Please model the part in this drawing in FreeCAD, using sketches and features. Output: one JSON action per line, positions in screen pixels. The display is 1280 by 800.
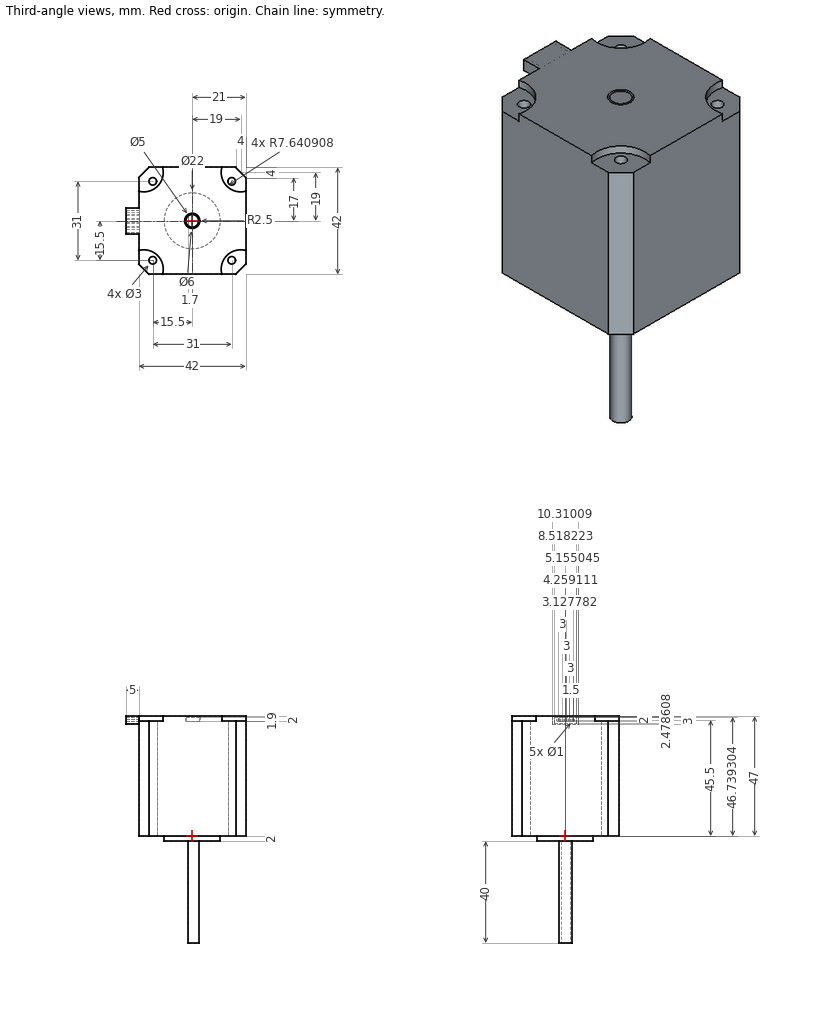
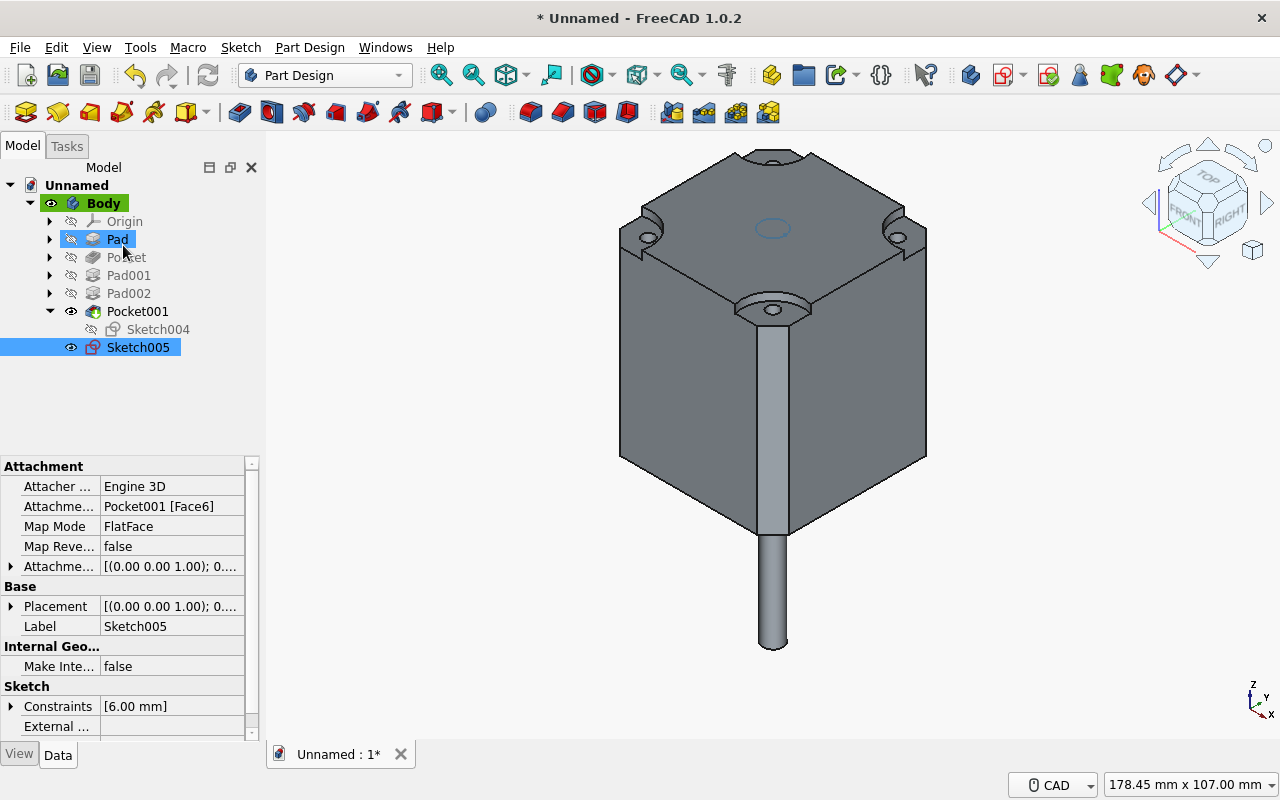
{"action": "left_click", "coordinate": [240, 112]}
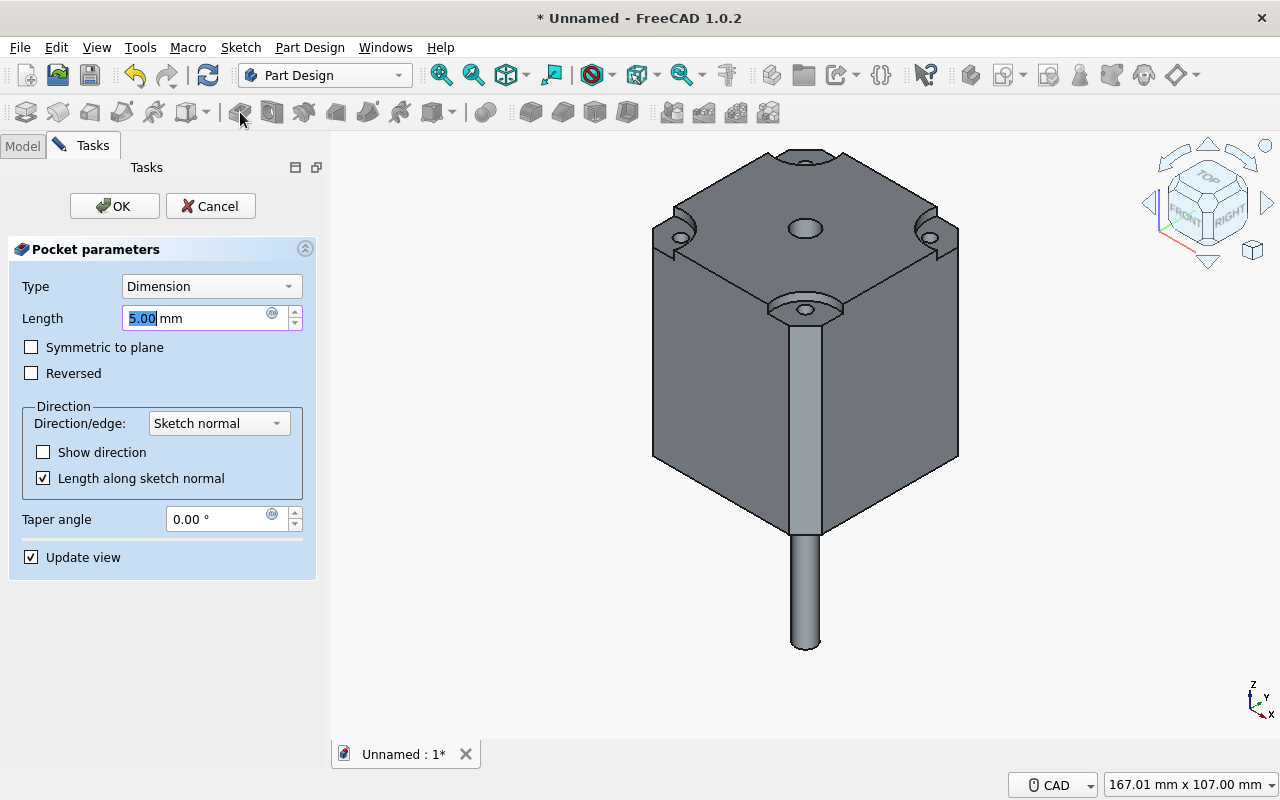
{"action": "type", "text": "2"}
{"action": "key", "text": "Tab"}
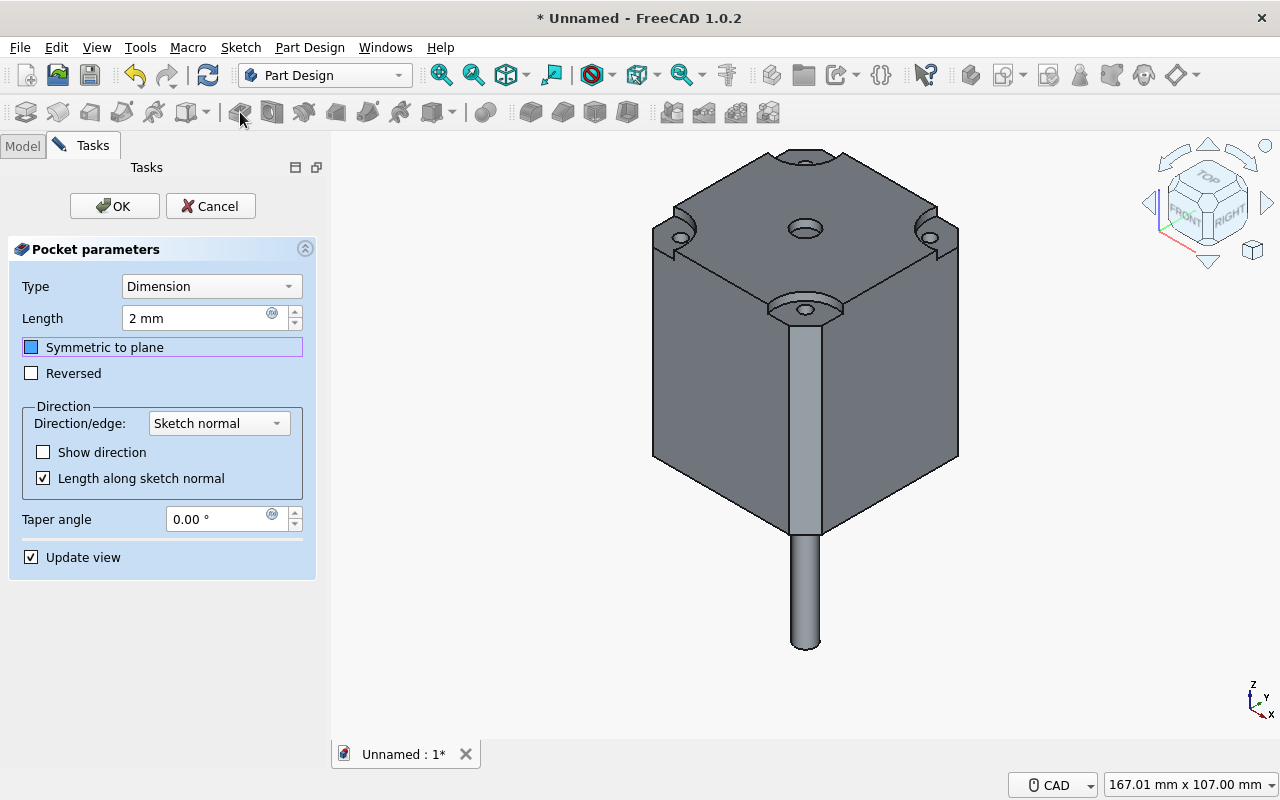
{"action": "left_click", "coordinate": [115, 206]}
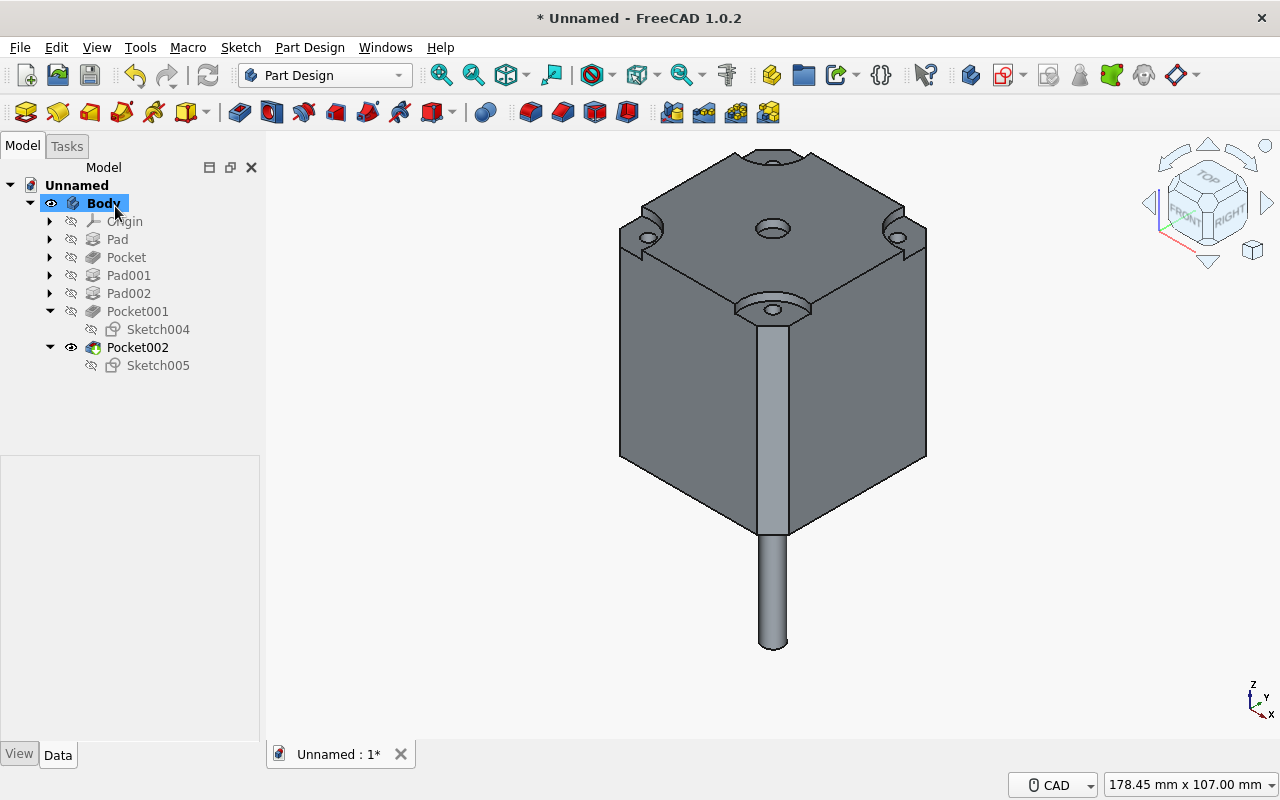
{"action": "left_click", "coordinate": [442, 76]}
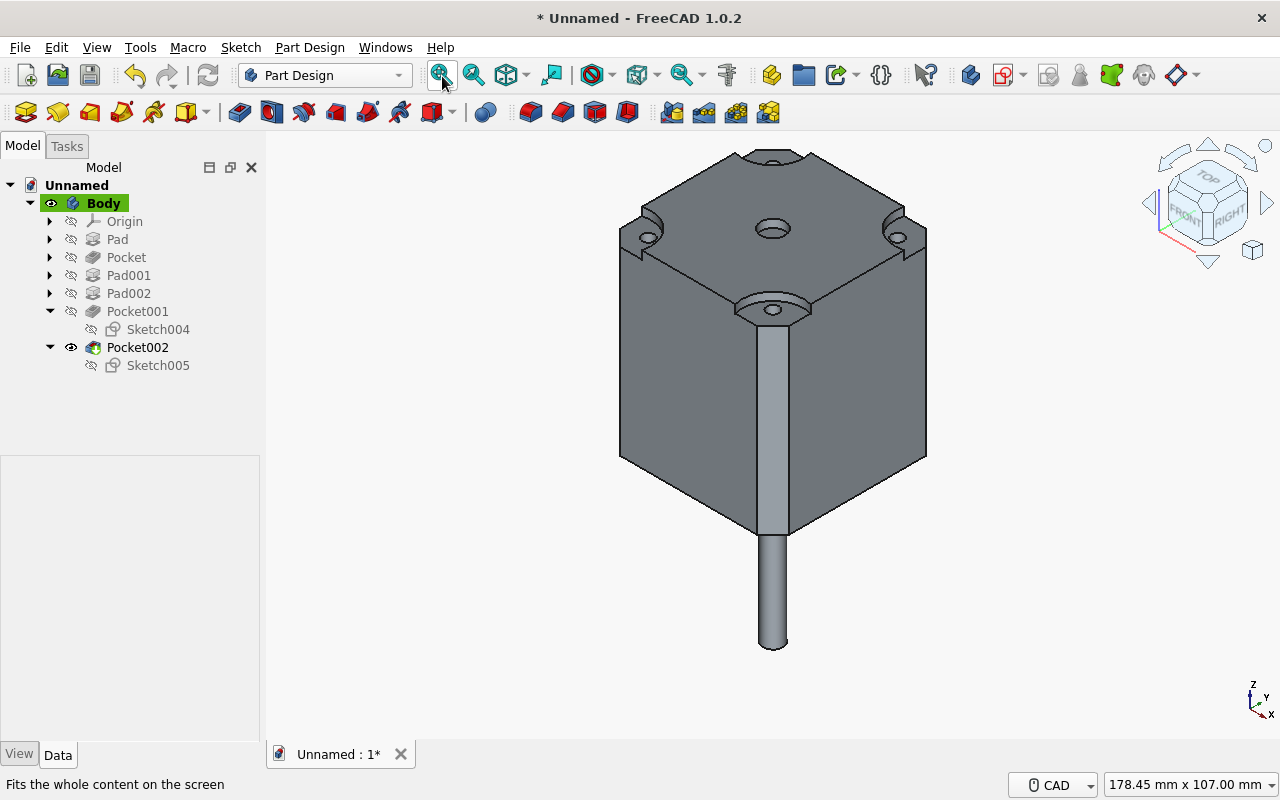
{"action": "left_click", "coordinate": [50, 221]}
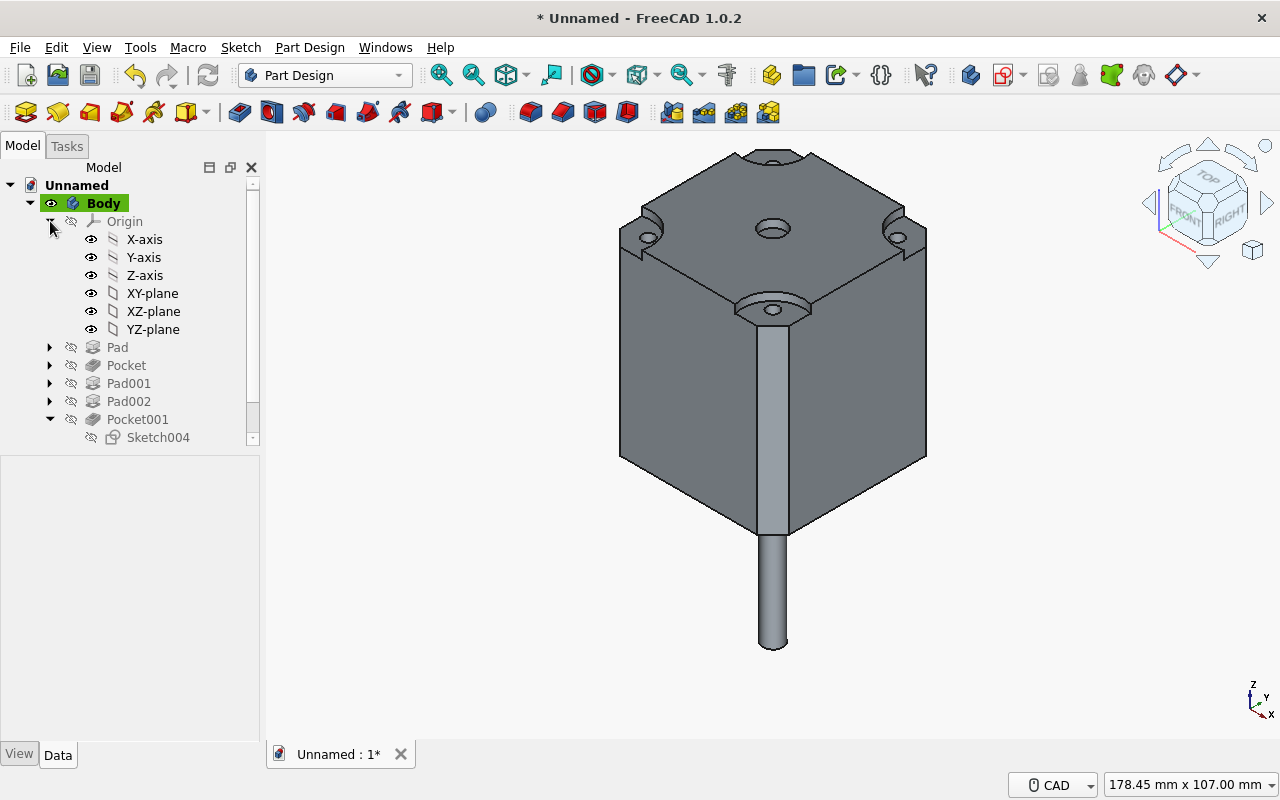
{"action": "left_click", "coordinate": [136, 293]}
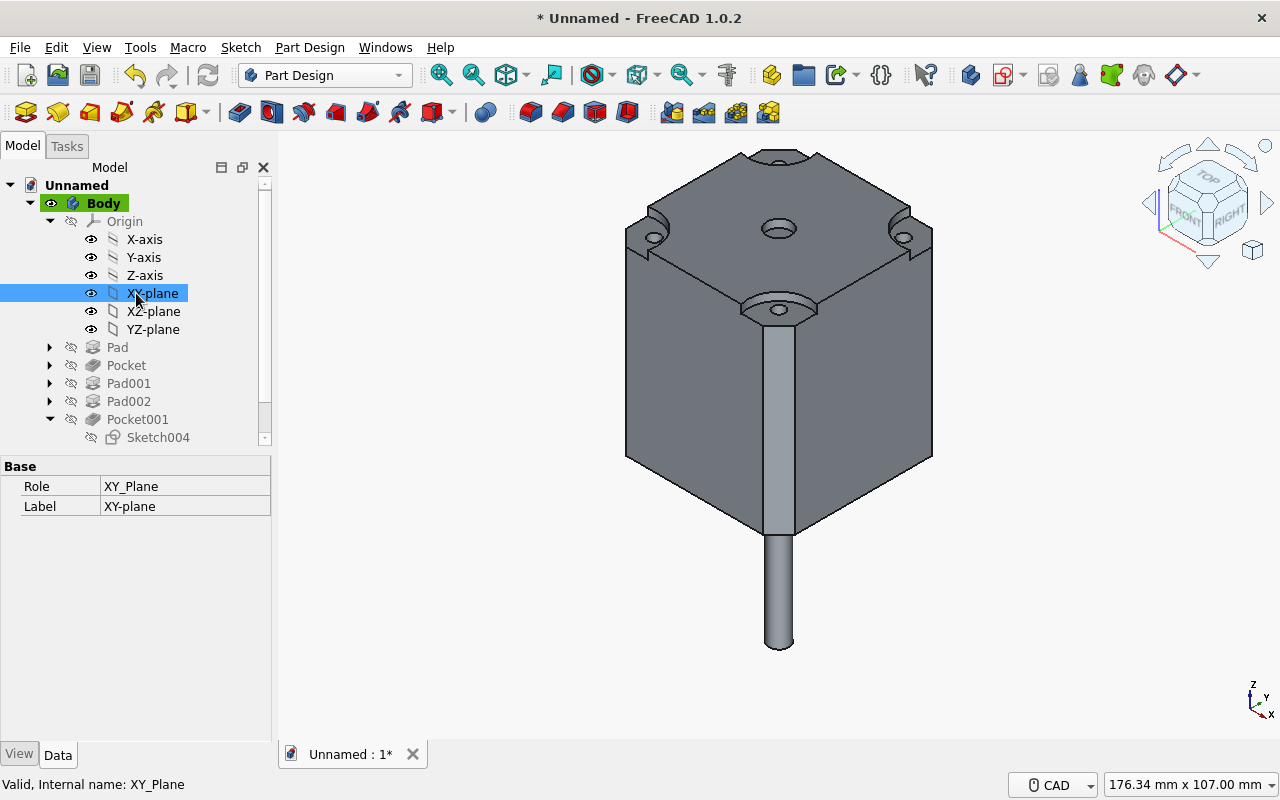
{"action": "left_click", "coordinate": [1176, 76]}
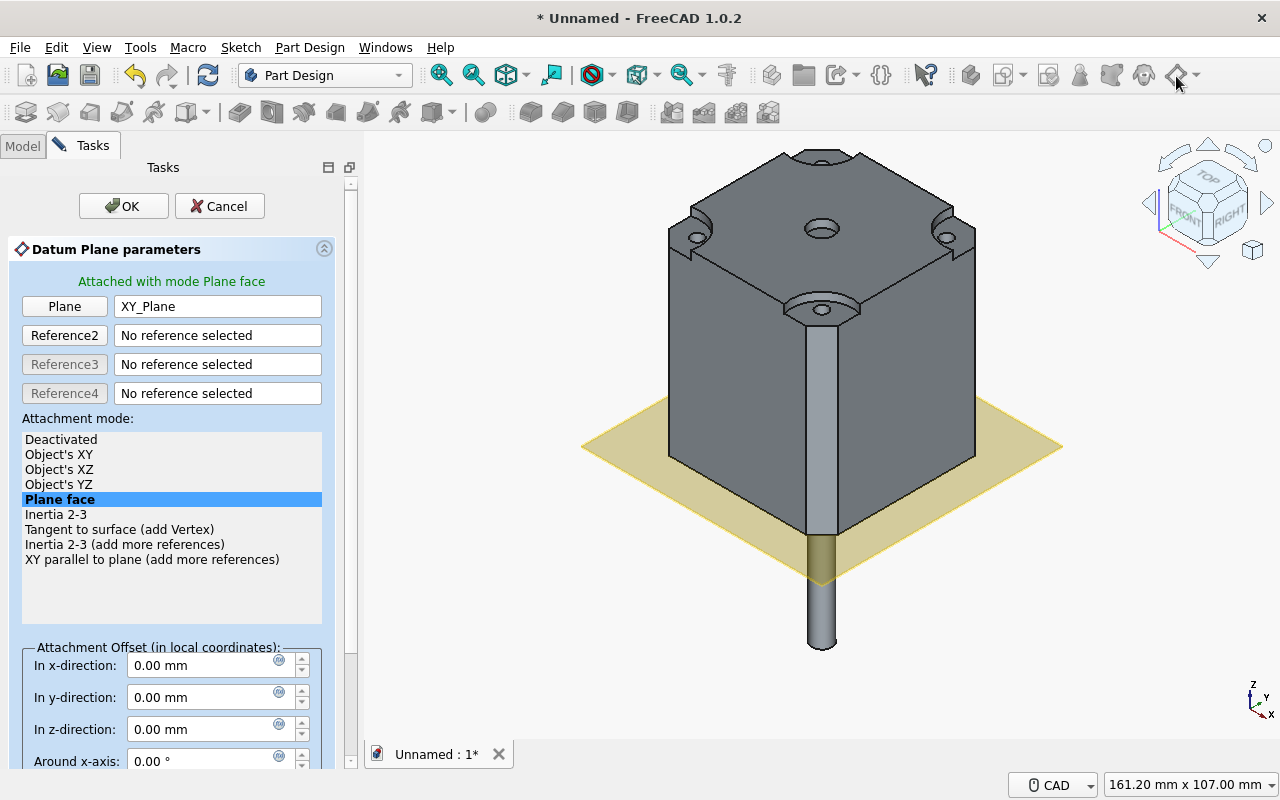
{"action": "triple_click", "coordinate": [210, 729]}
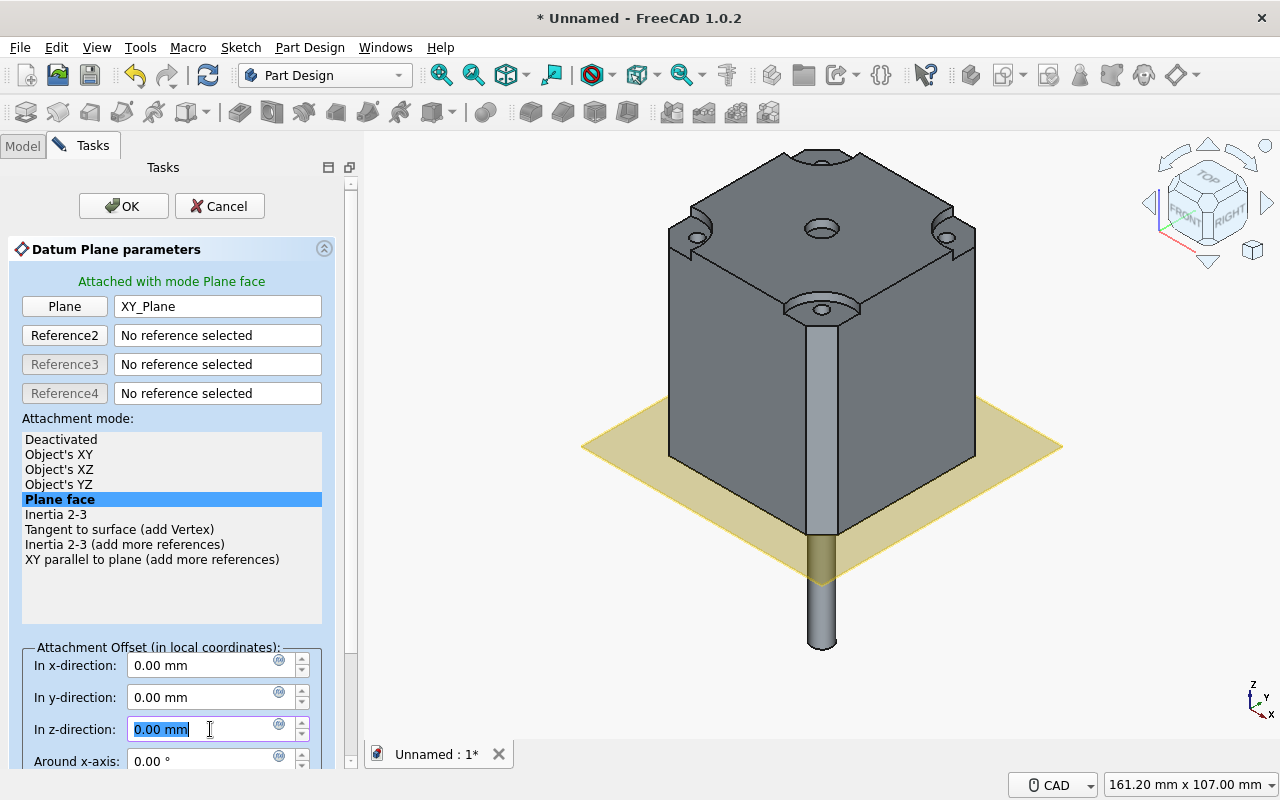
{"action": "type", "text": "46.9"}
{"action": "key", "text": "Tab"}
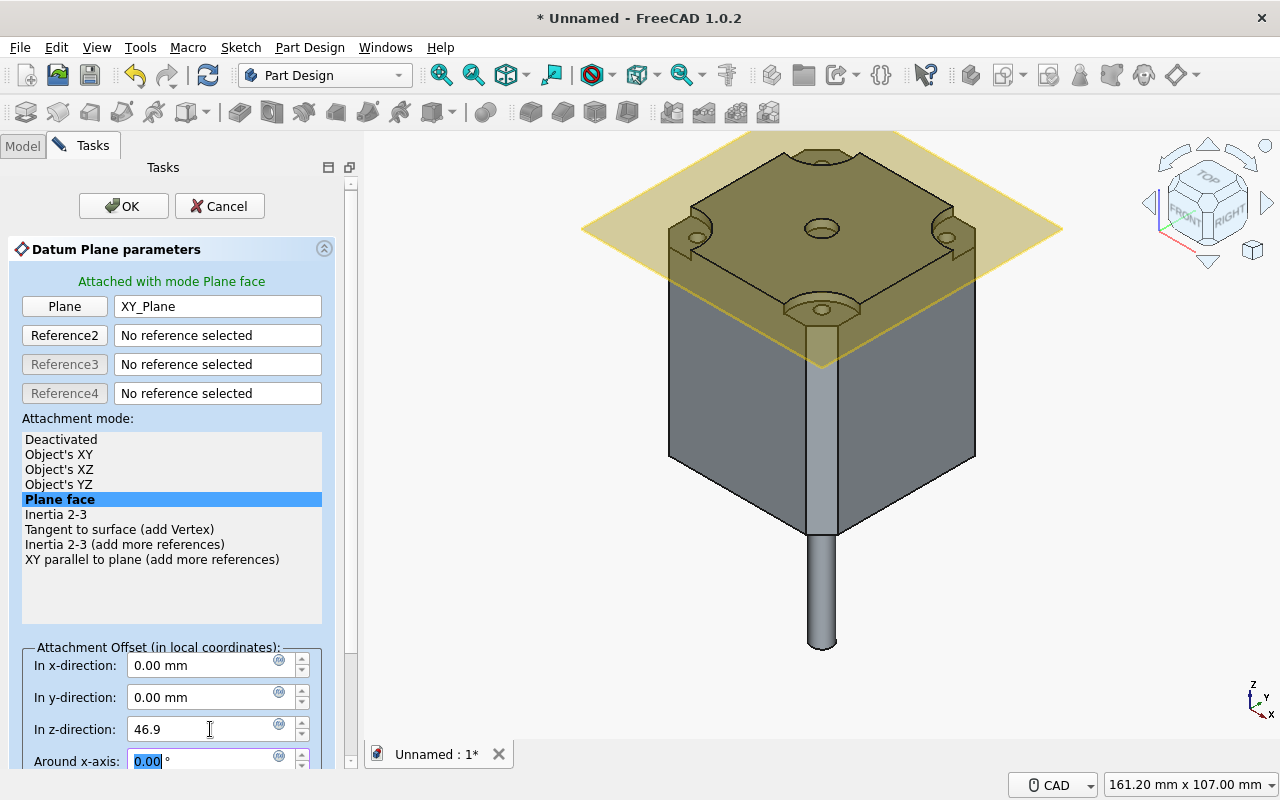
{"action": "left_click", "coordinate": [124, 206]}